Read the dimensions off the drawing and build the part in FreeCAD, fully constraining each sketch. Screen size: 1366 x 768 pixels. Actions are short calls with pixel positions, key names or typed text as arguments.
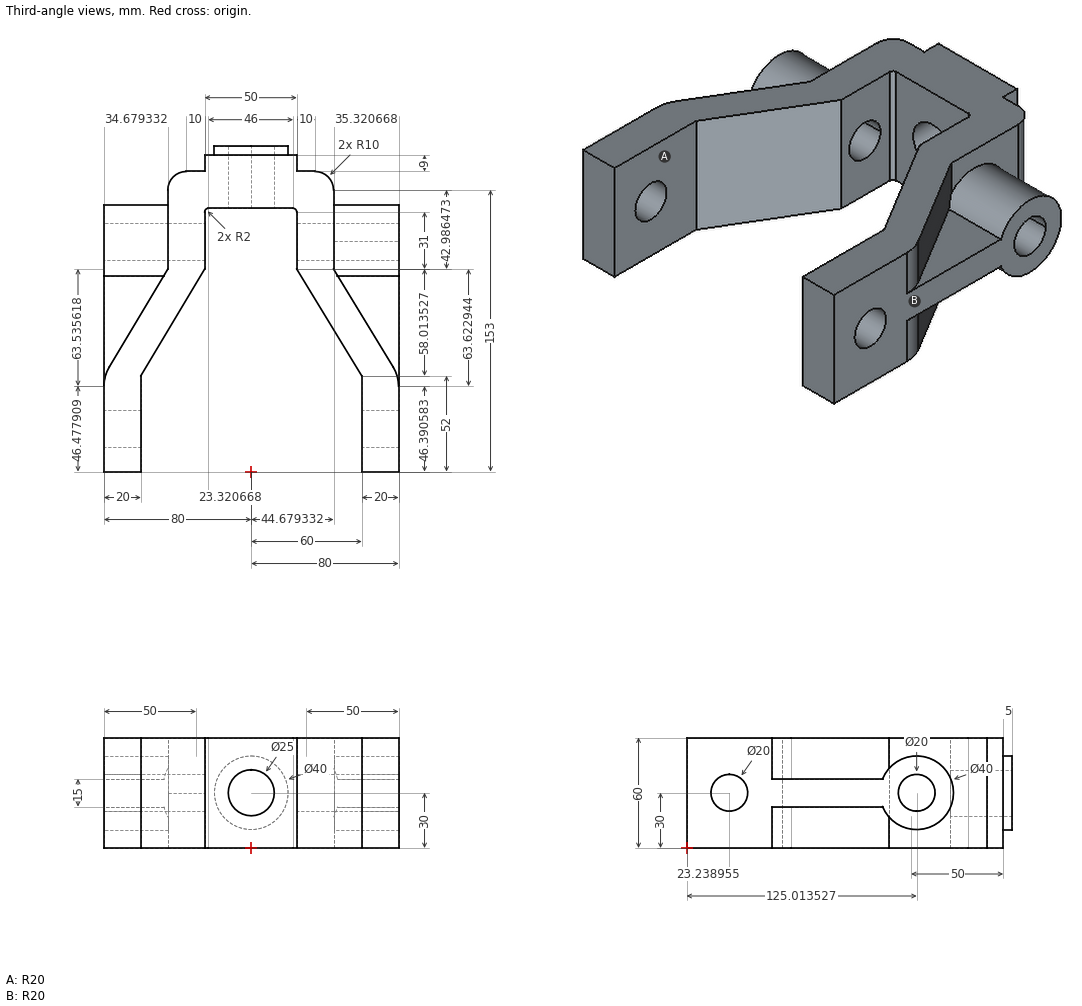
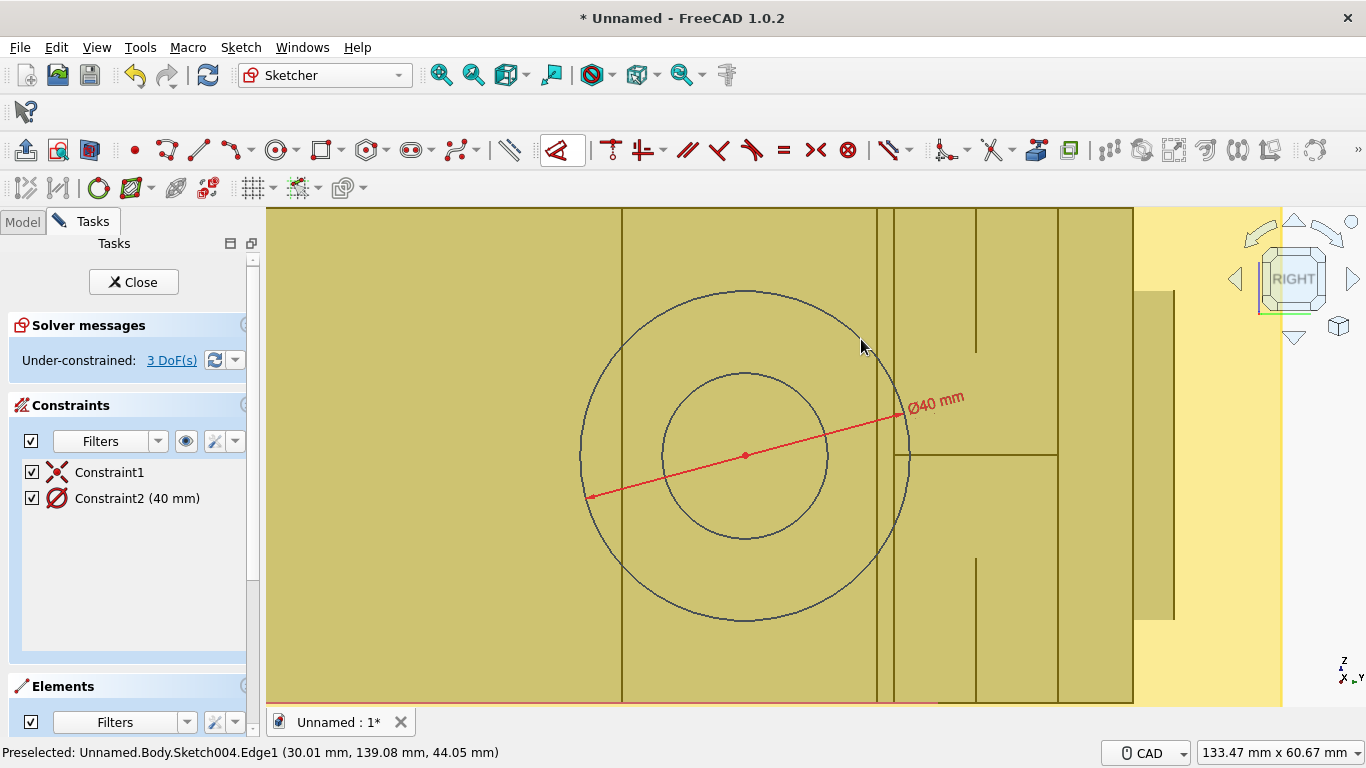
click(803, 397)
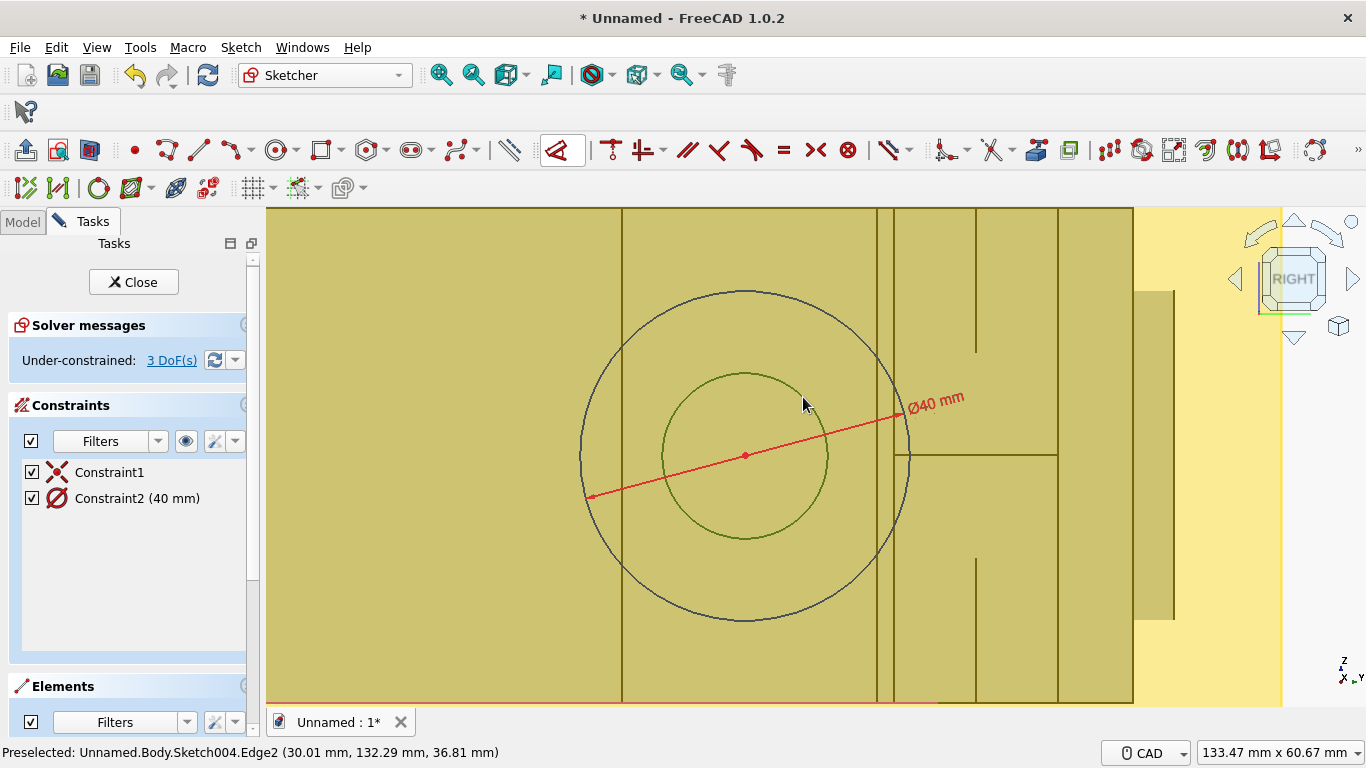
key(k)
key(o)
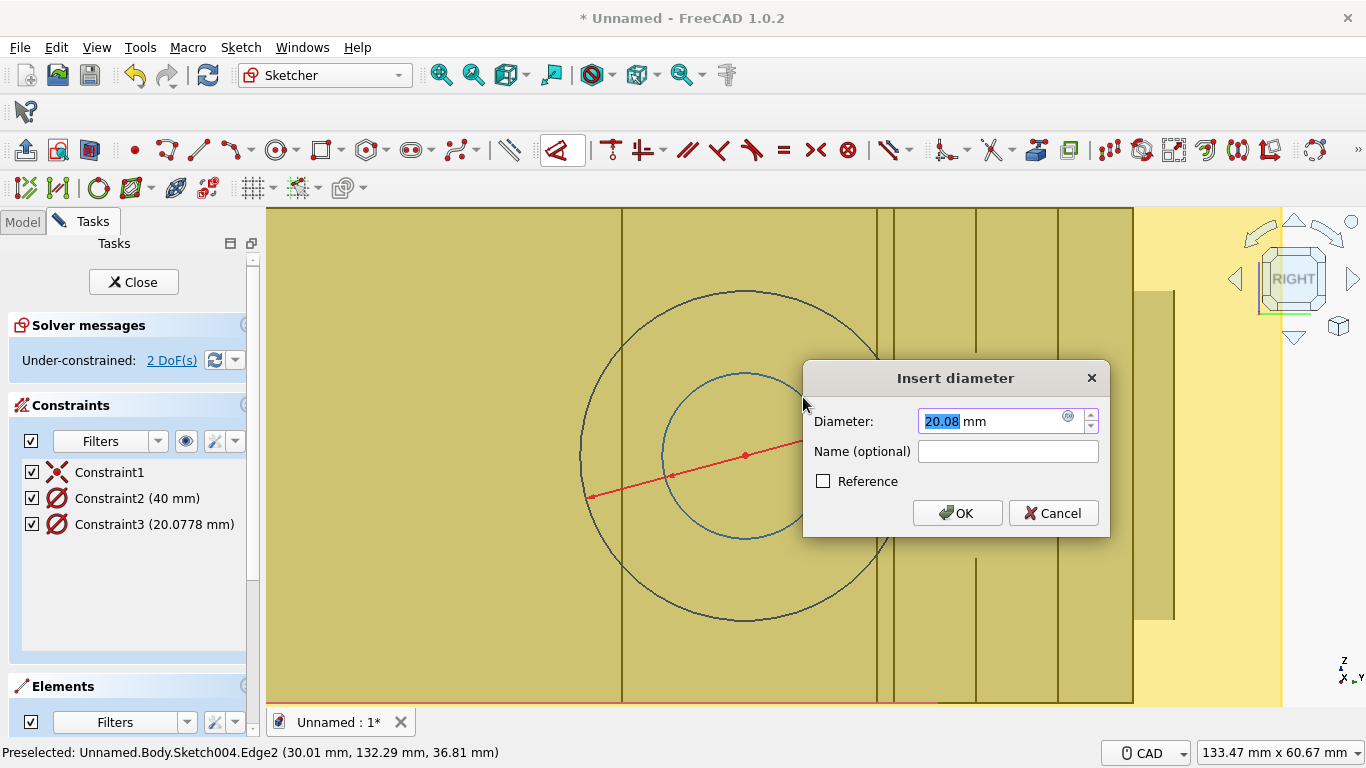
text(20)
key(Return)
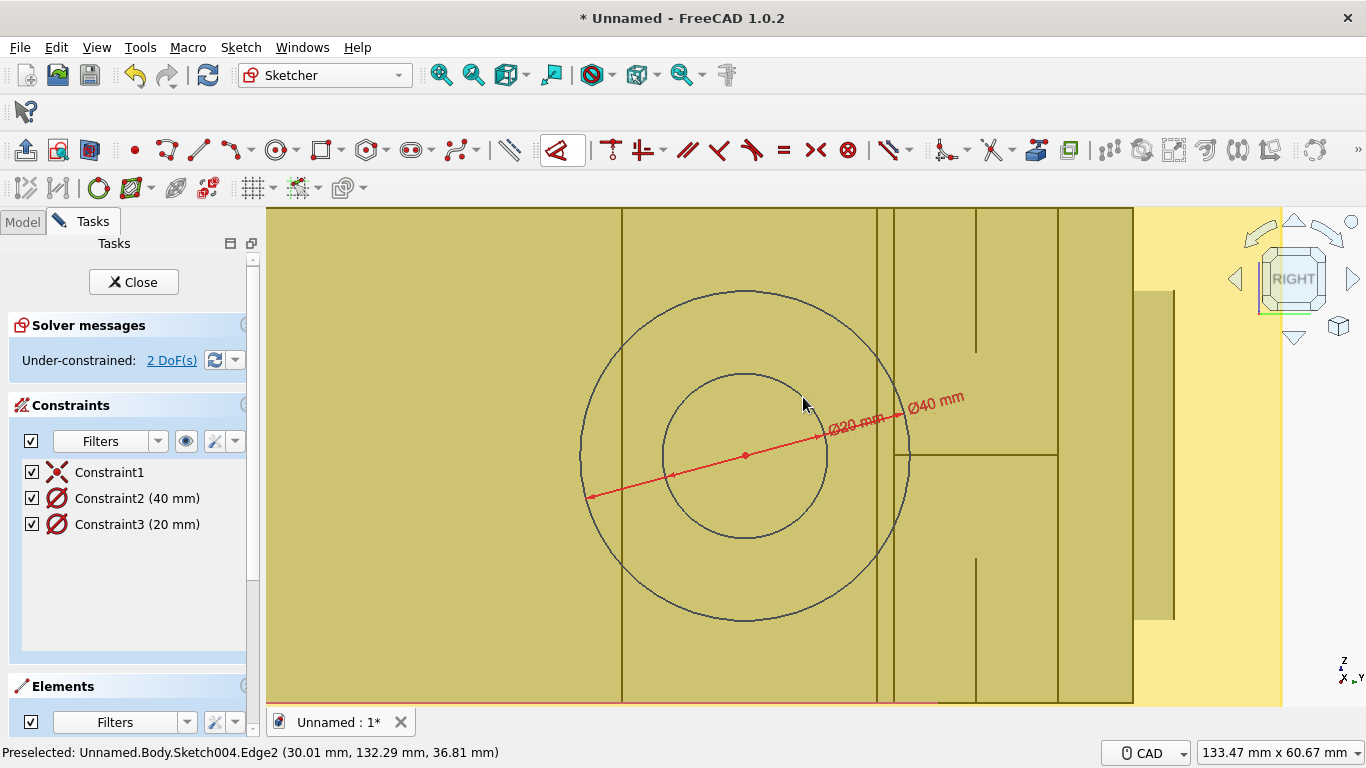
click(745, 456)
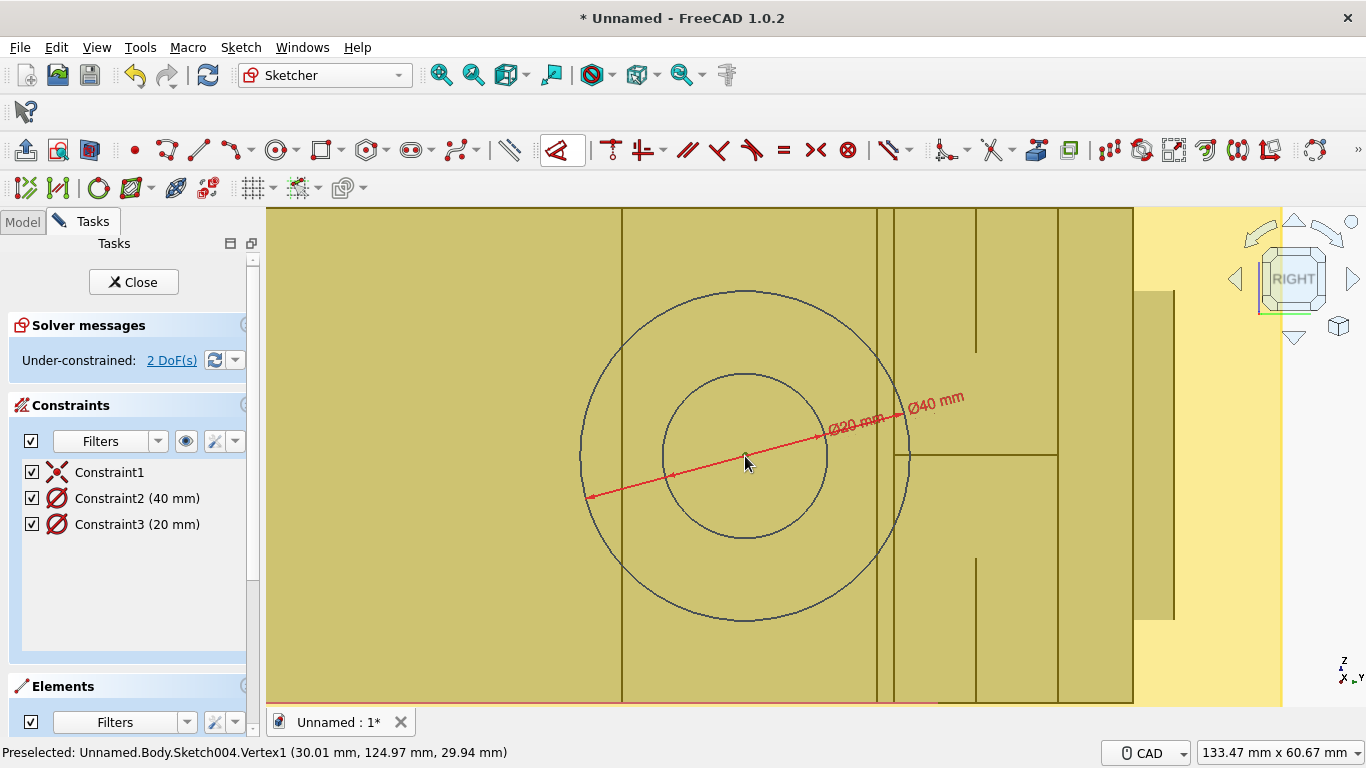
key(i)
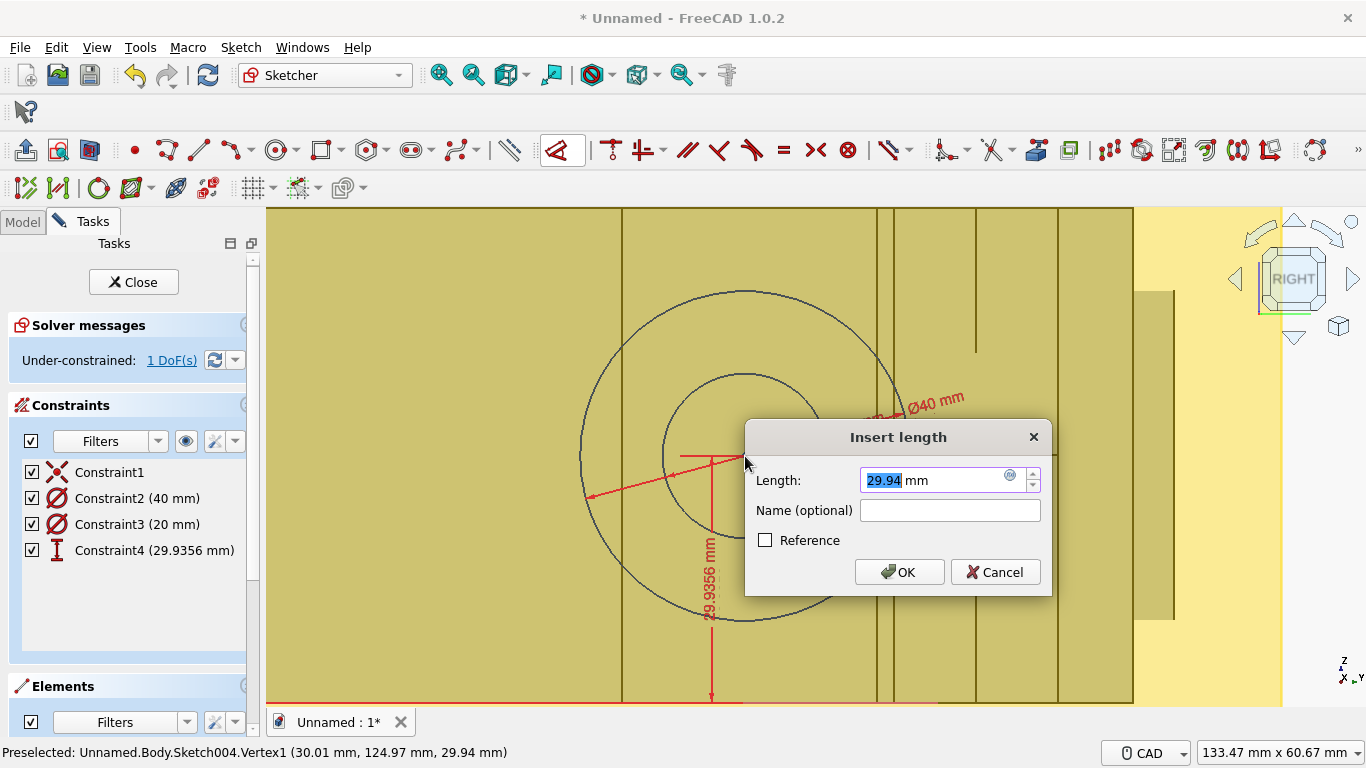
text(30)
key(Return)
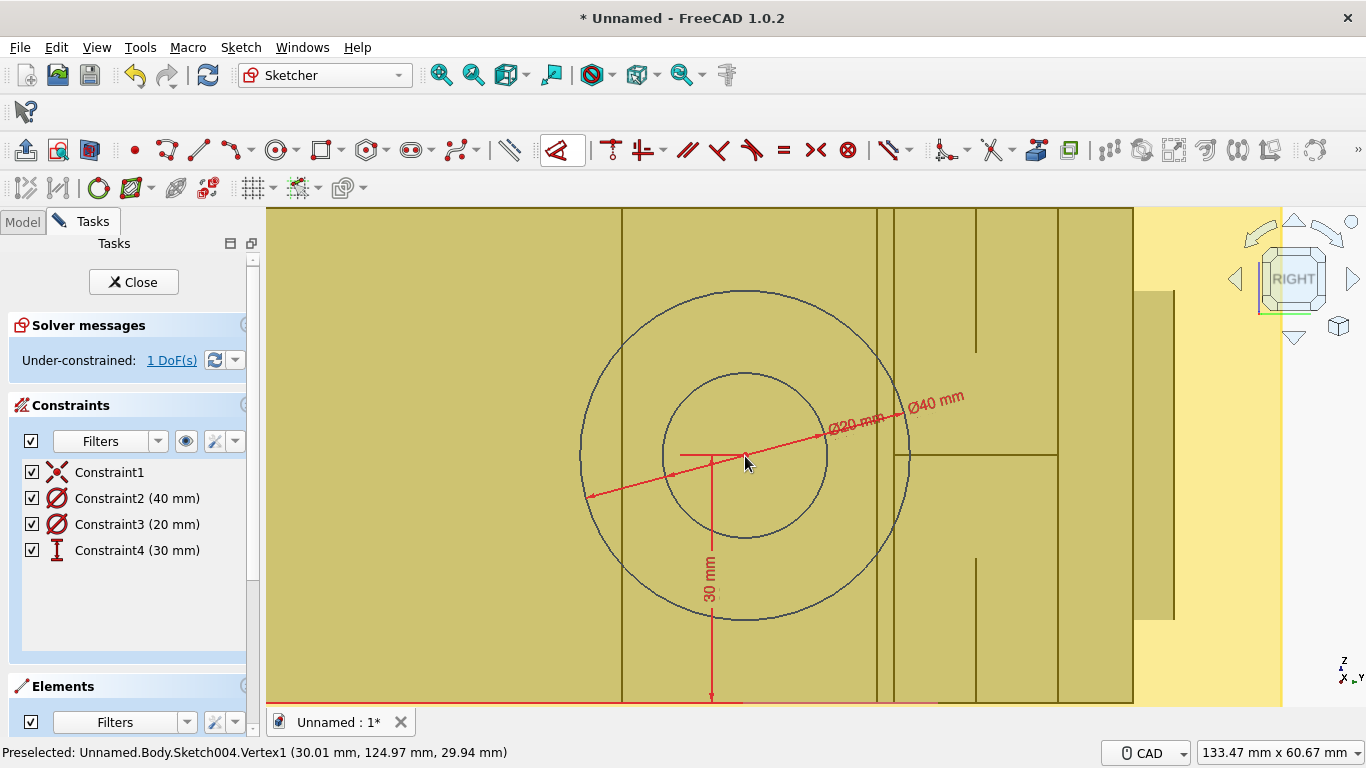
click(745, 455)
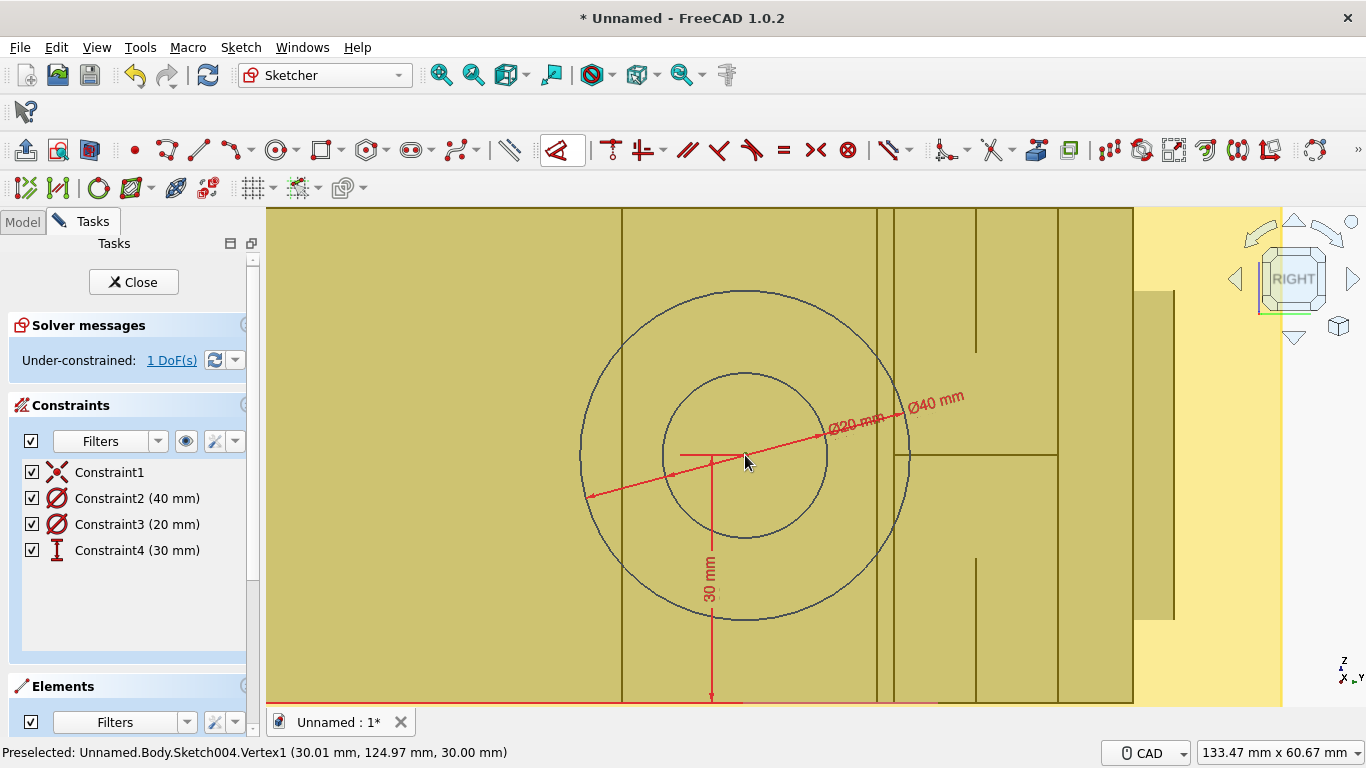
key(l)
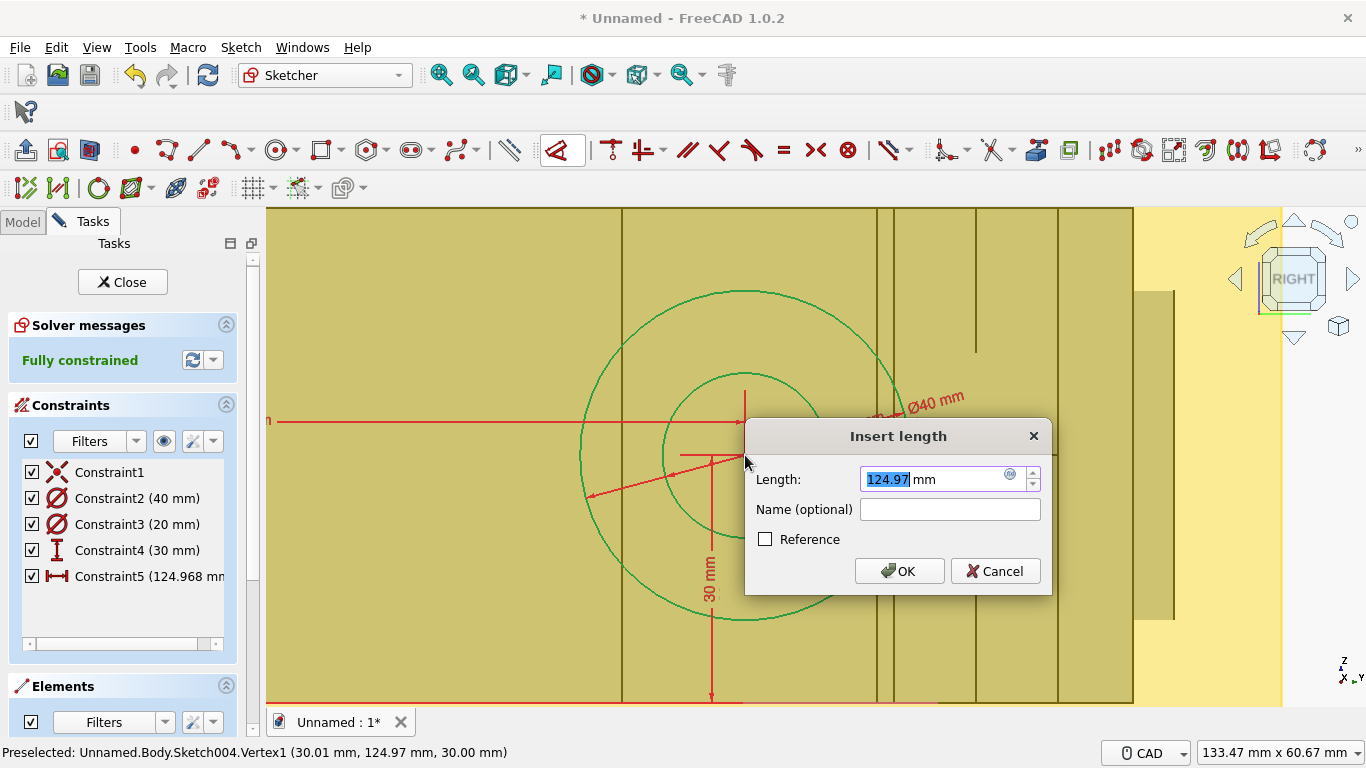
text(125.013527)
key(Return)